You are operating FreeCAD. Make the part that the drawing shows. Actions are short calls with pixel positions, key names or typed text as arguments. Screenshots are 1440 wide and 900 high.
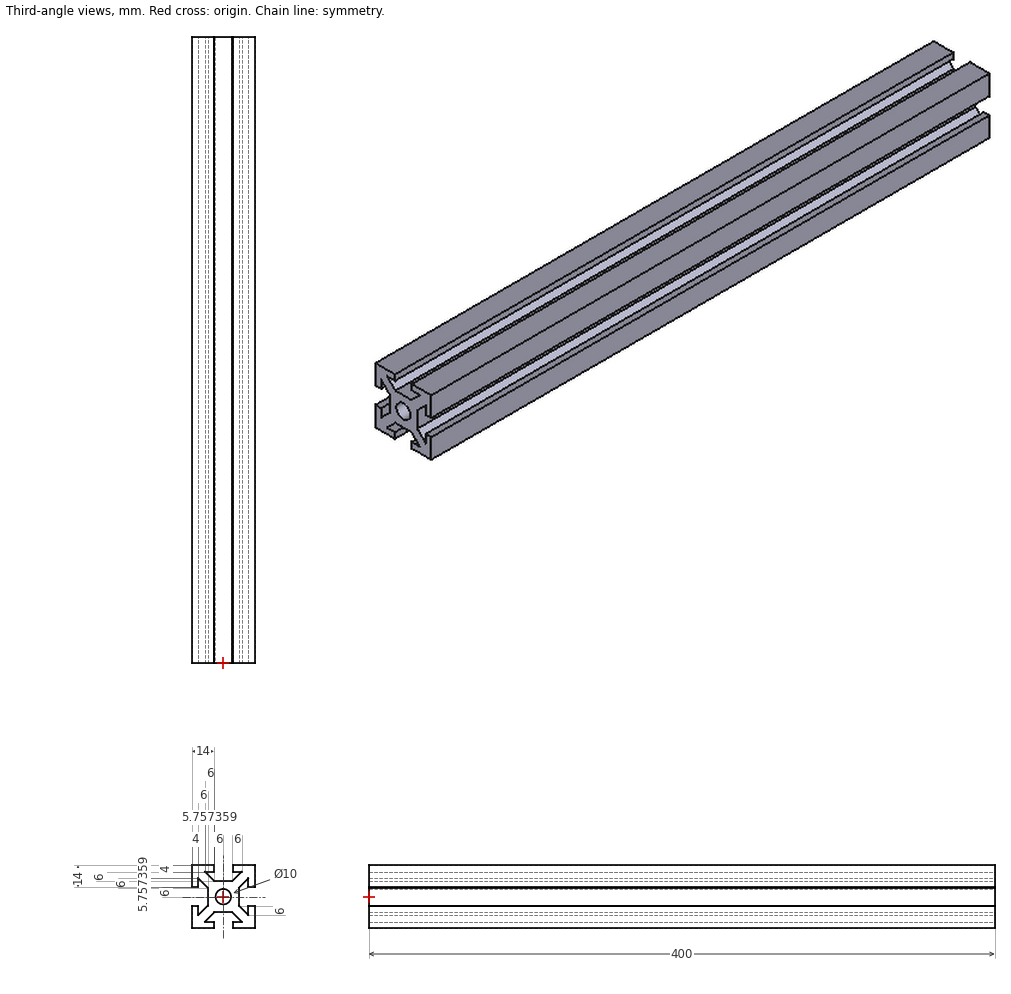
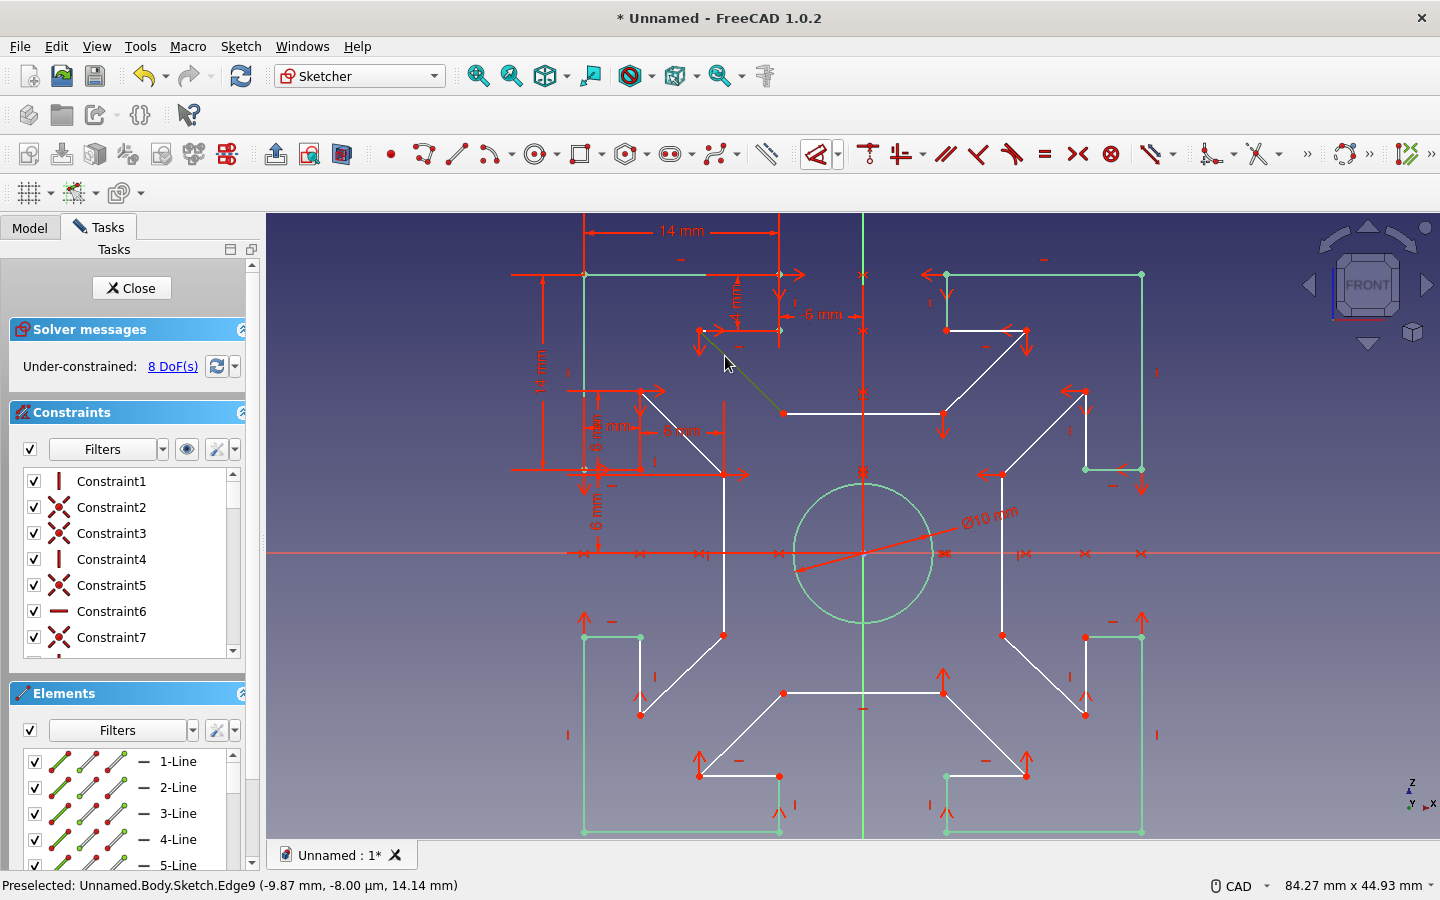
click(838, 154)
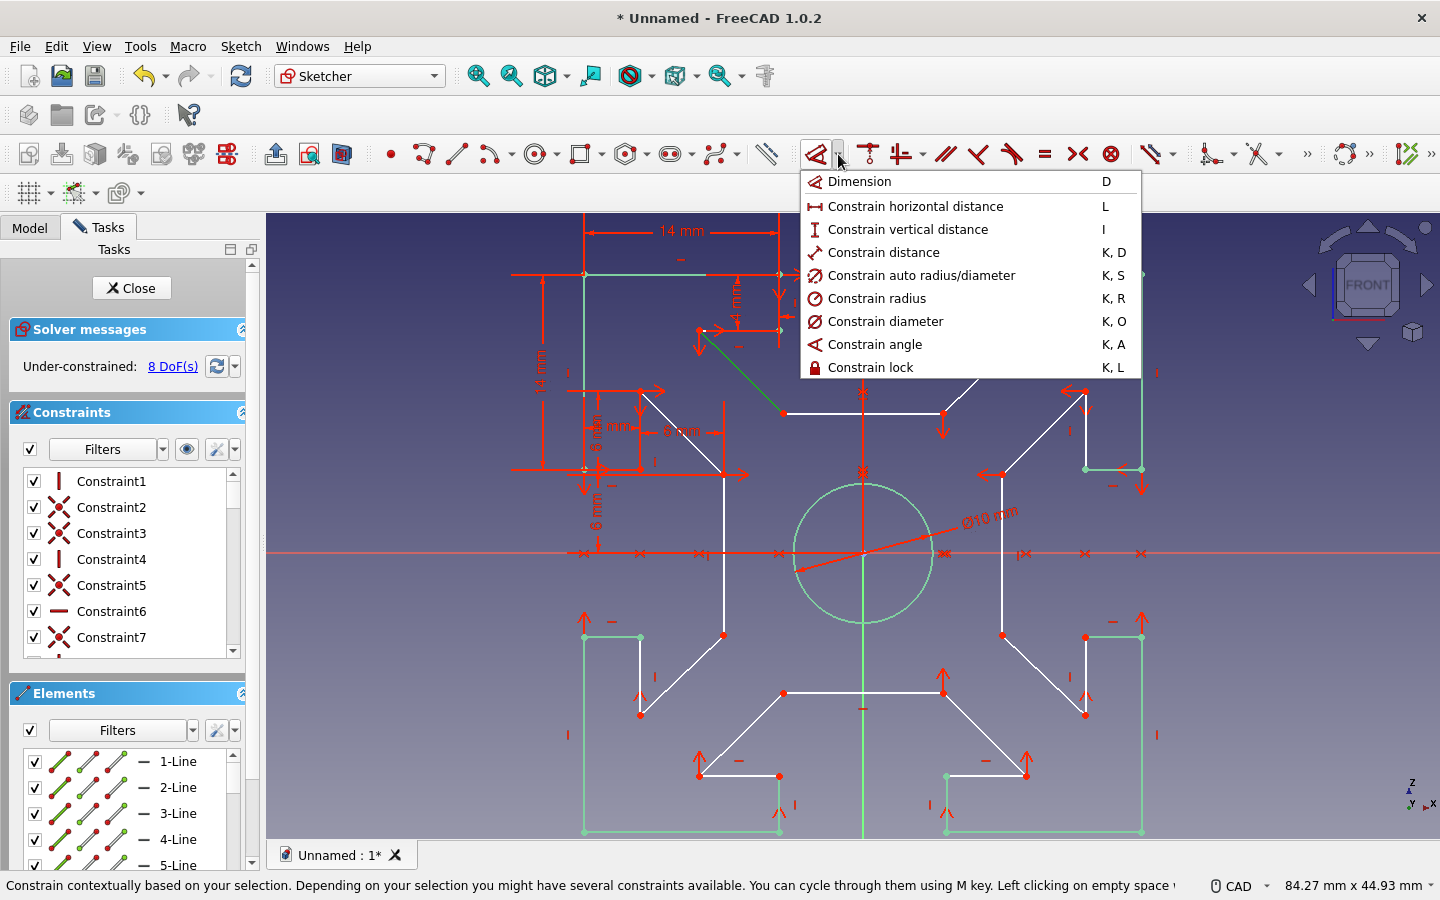
click(971, 206)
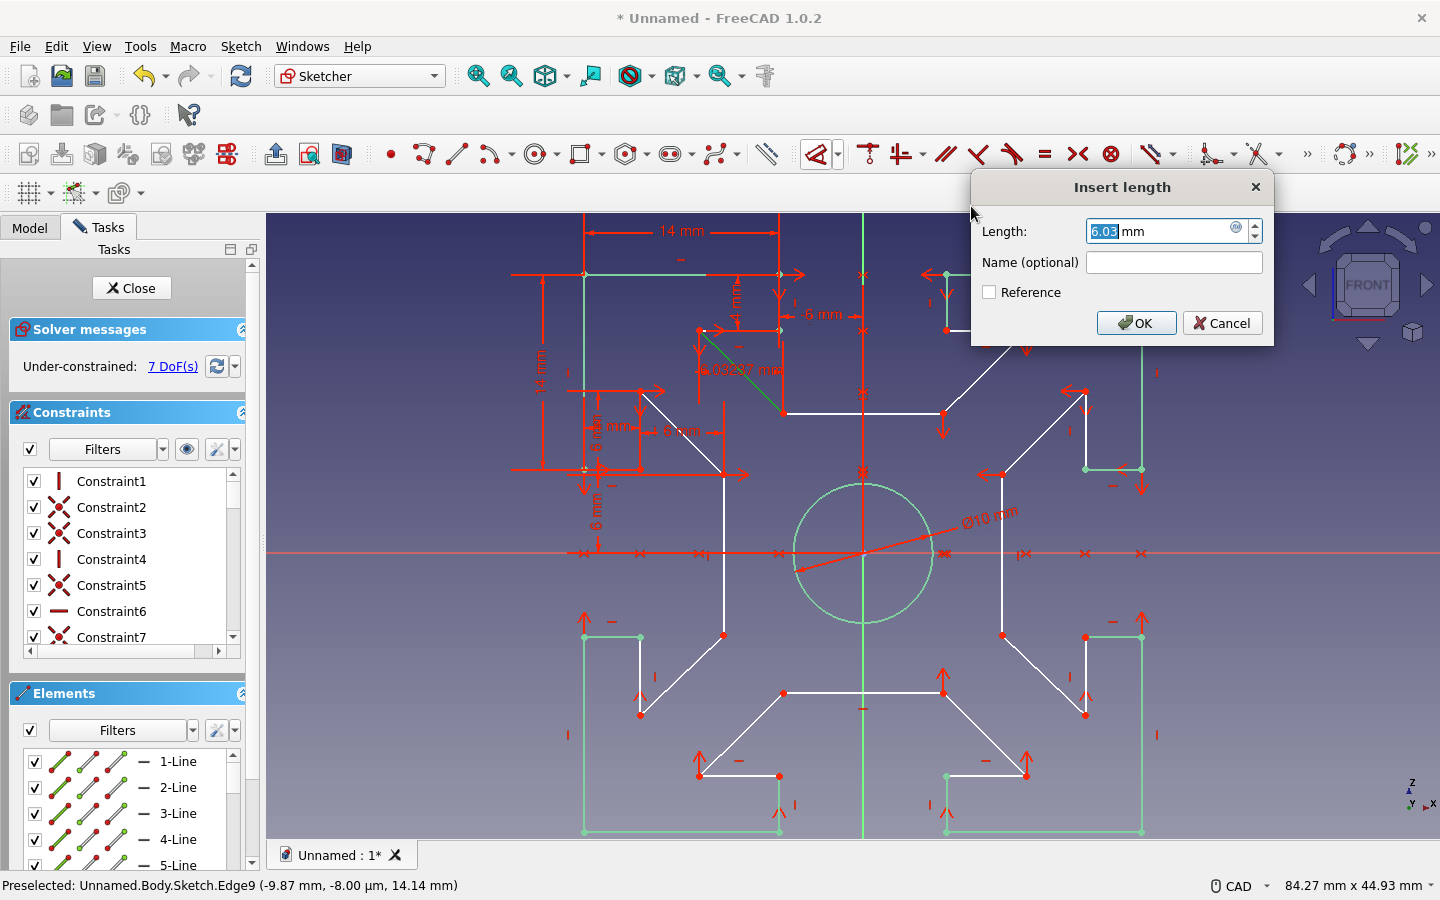
text(6)
key(Return)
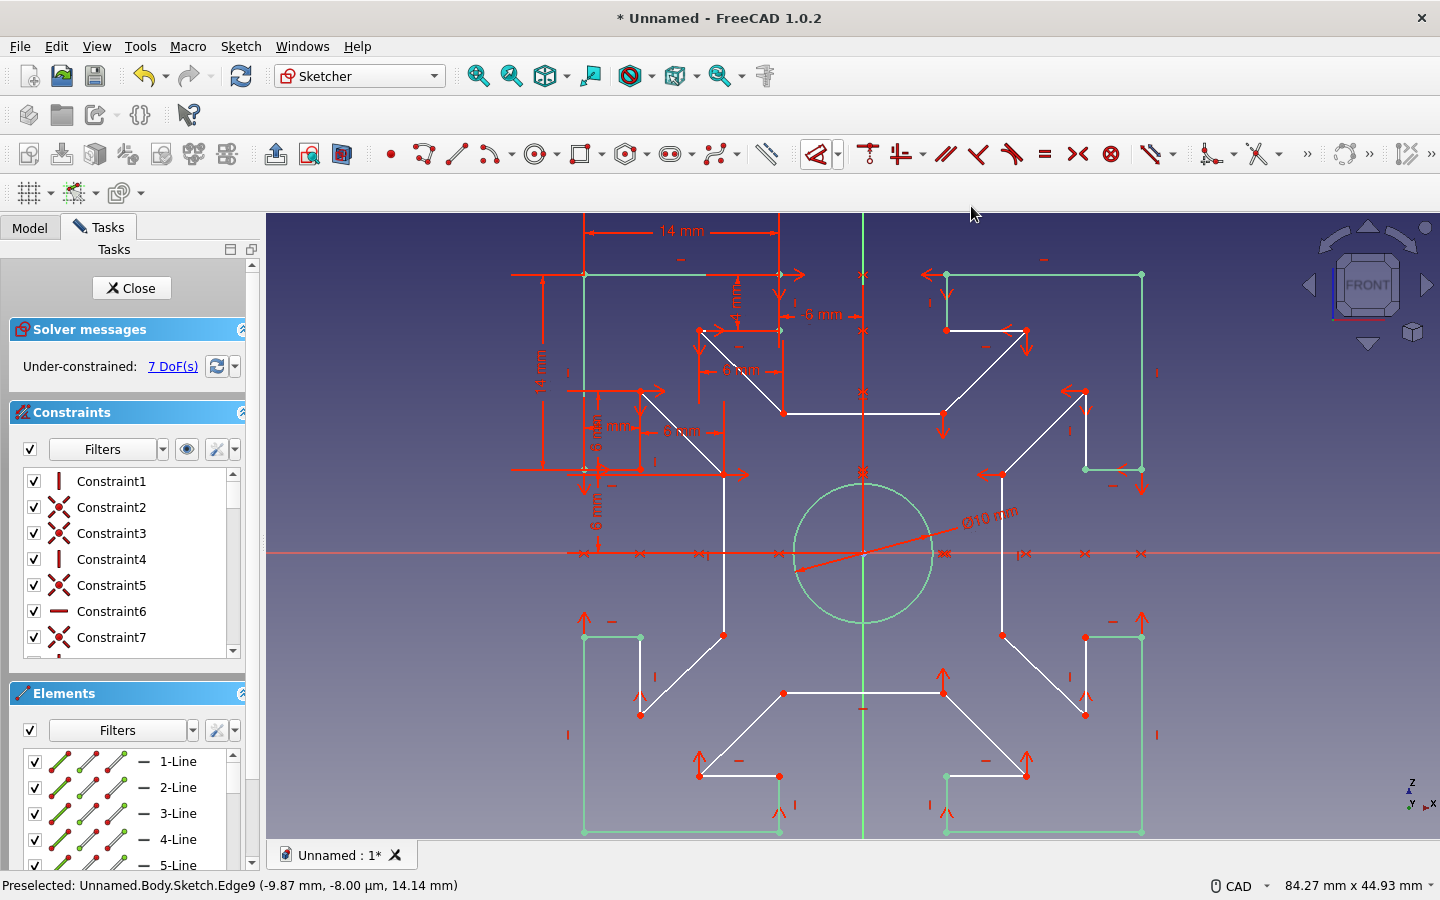
click(725, 356)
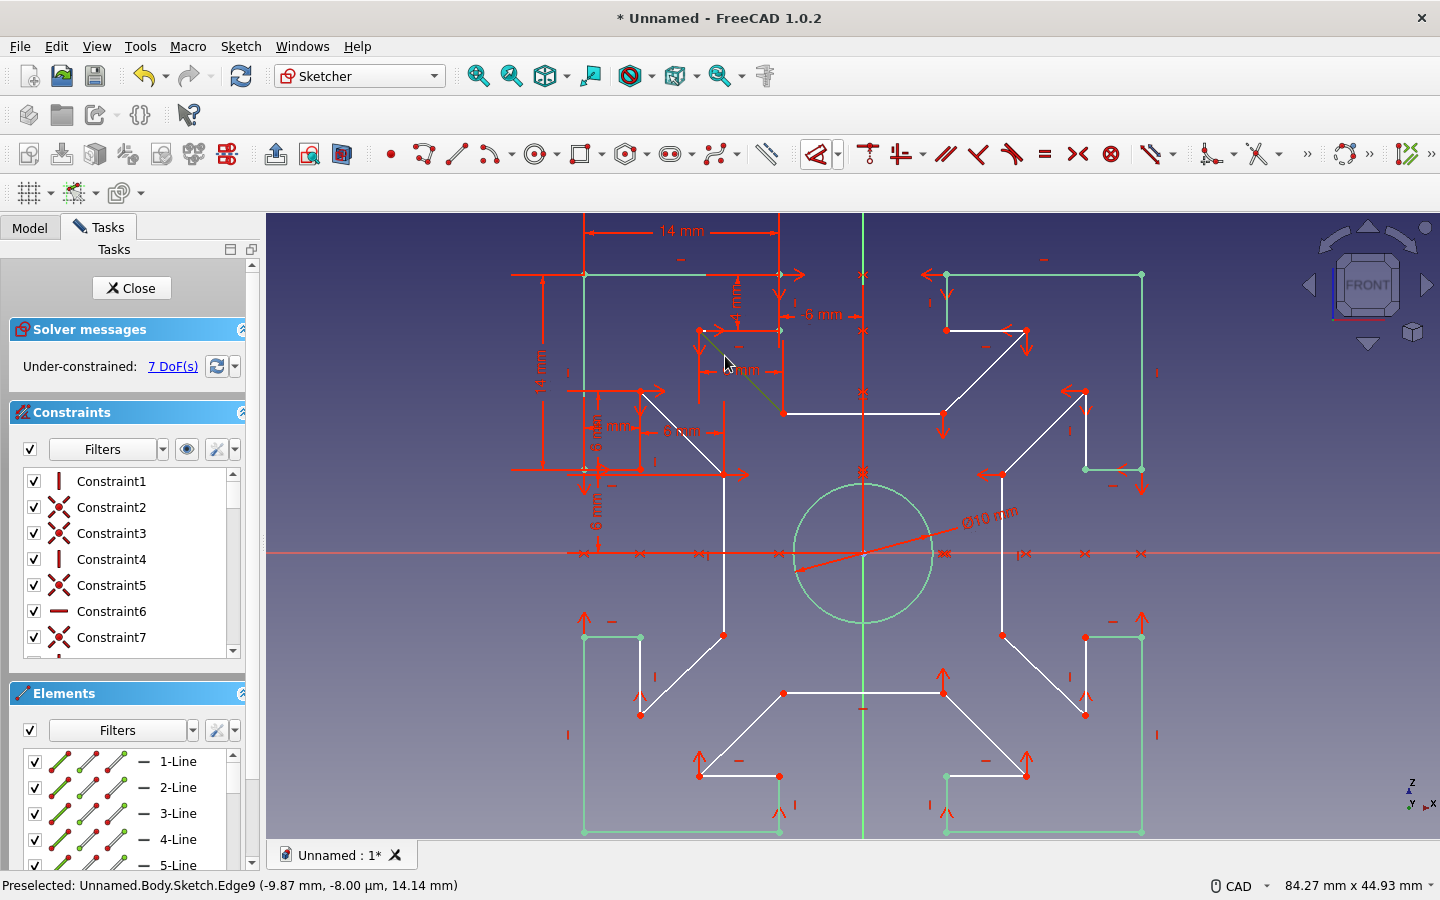
key(i)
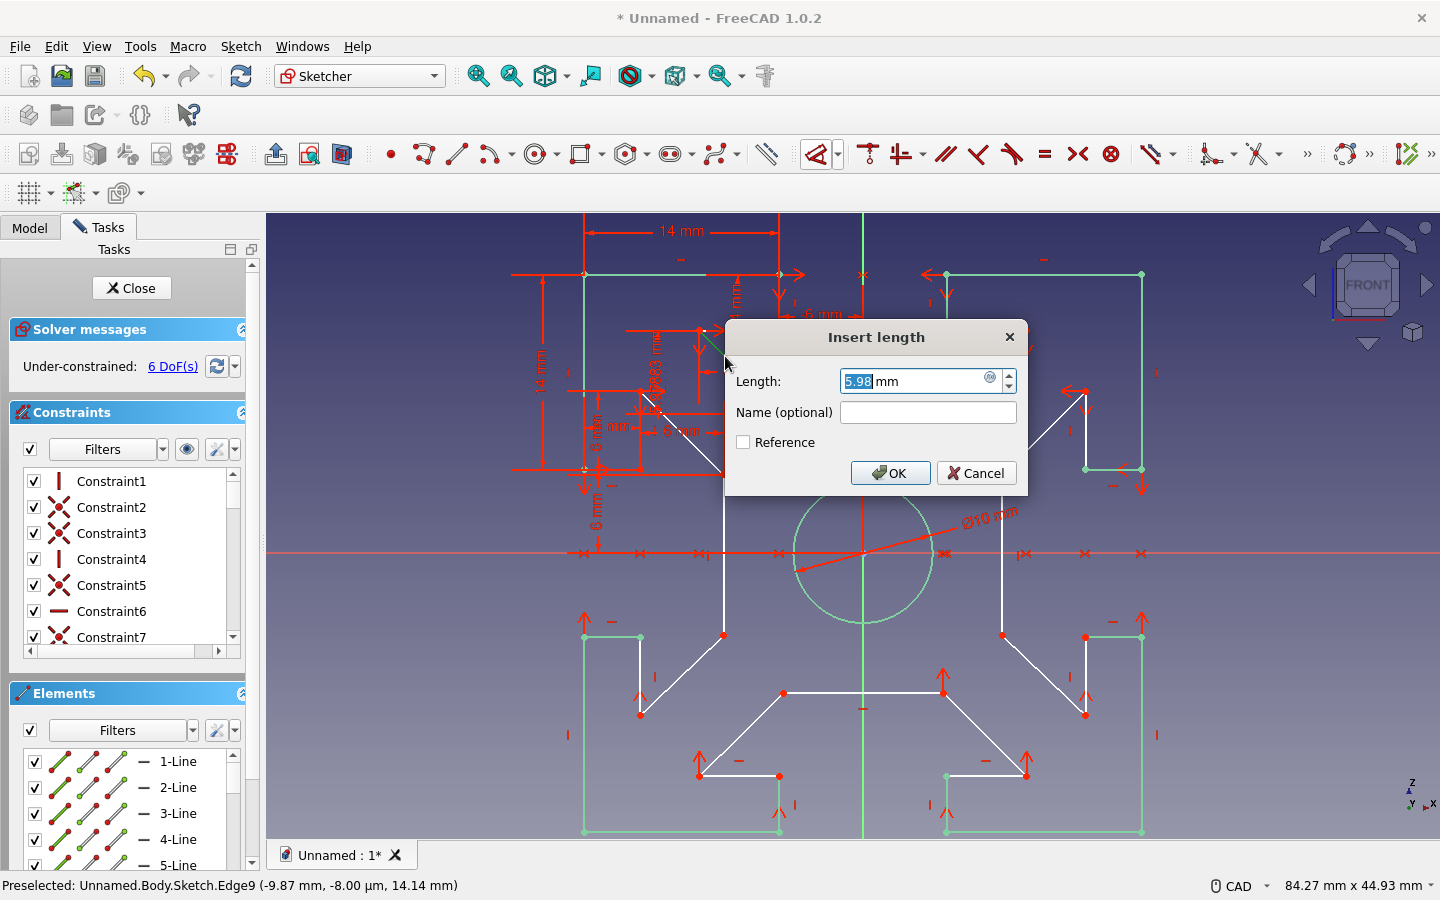
text(6)
key(Return)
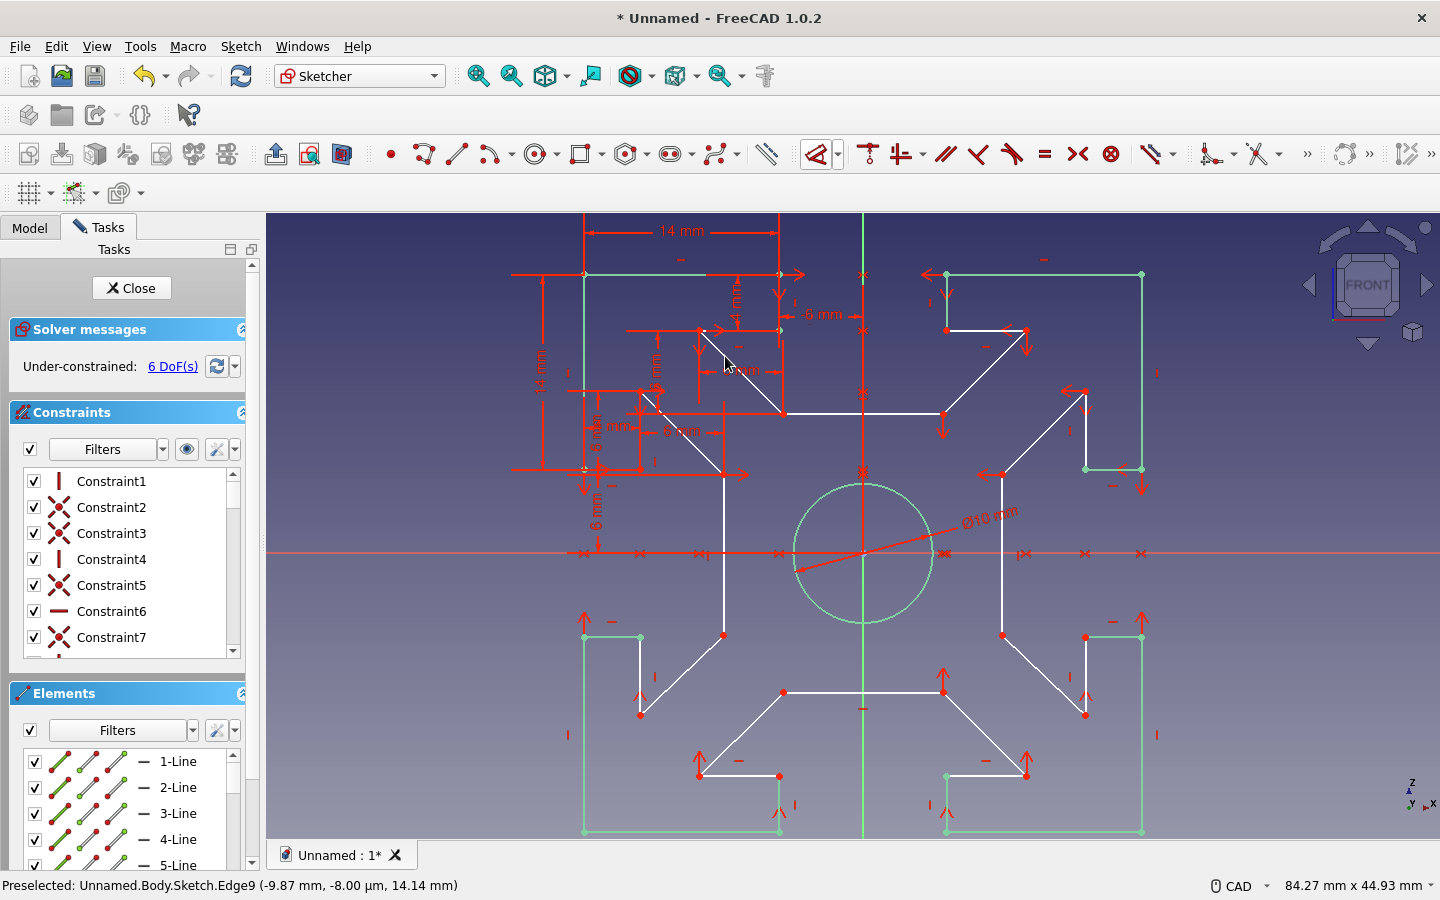
click(968, 389)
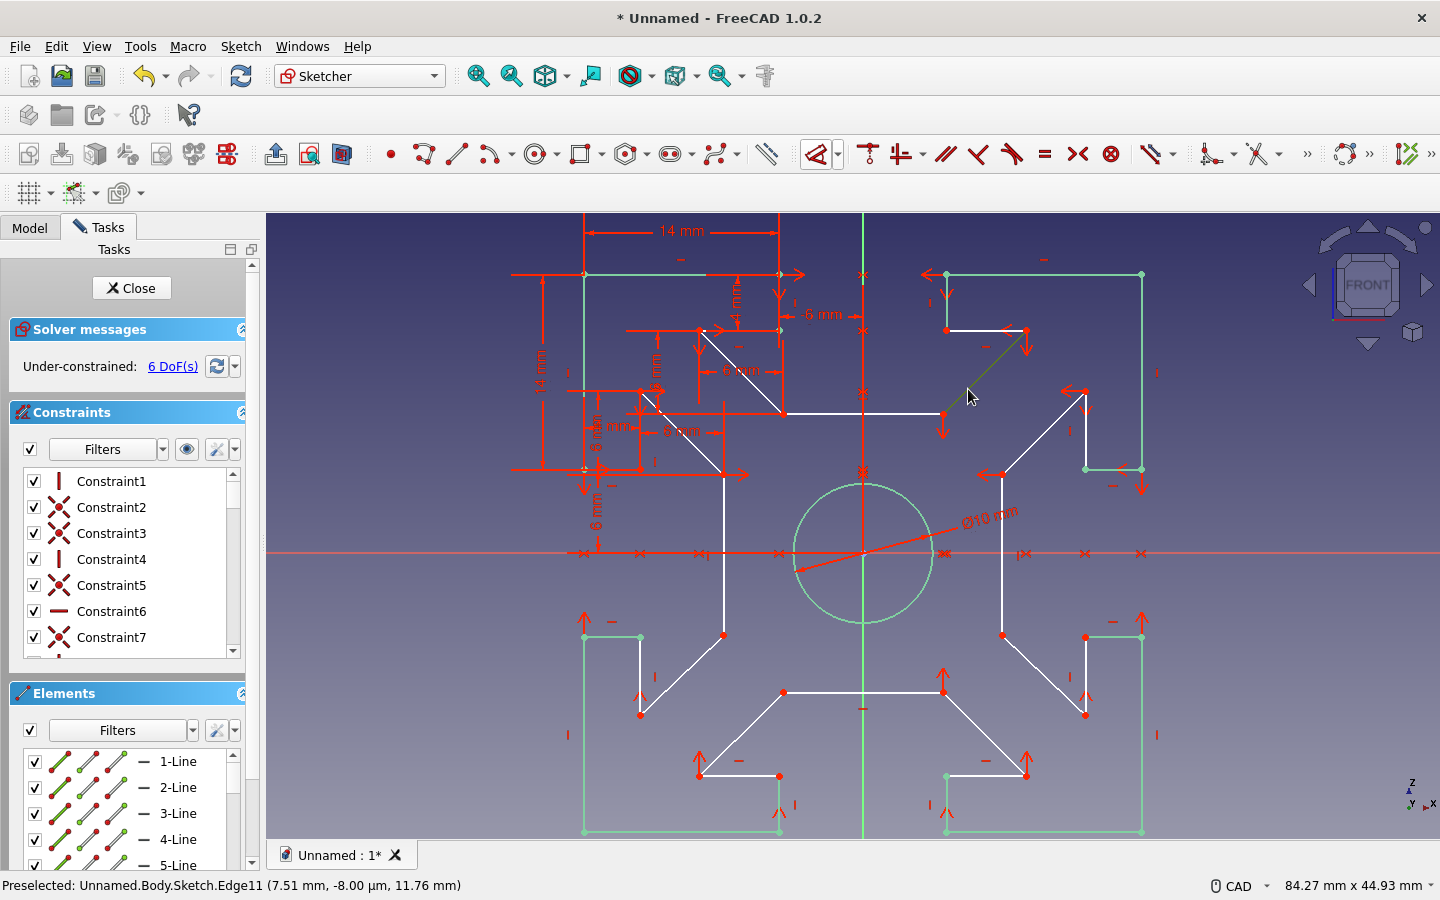
click(838, 154)